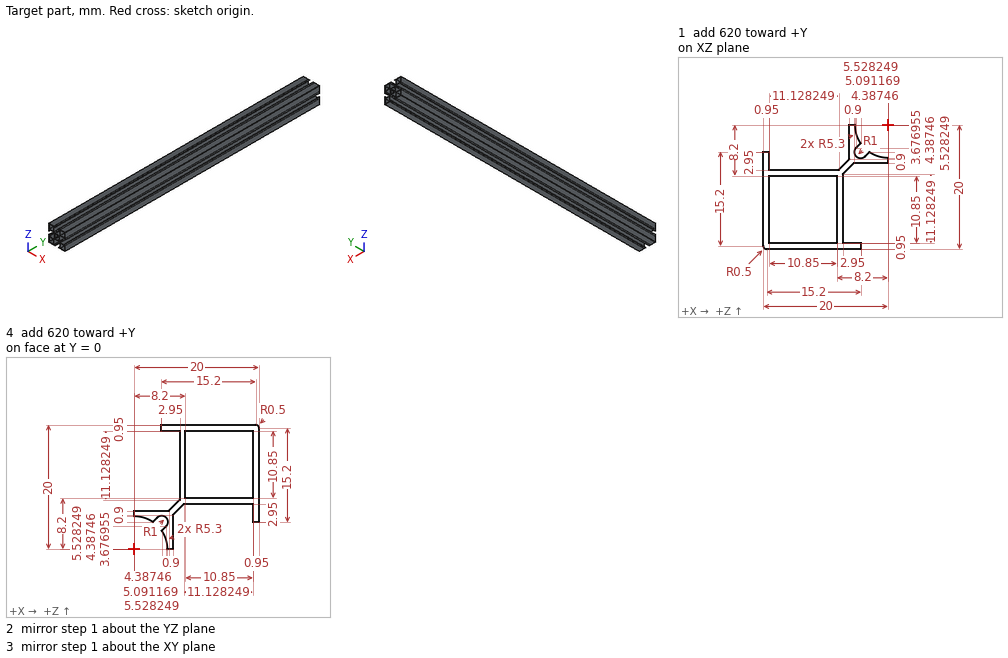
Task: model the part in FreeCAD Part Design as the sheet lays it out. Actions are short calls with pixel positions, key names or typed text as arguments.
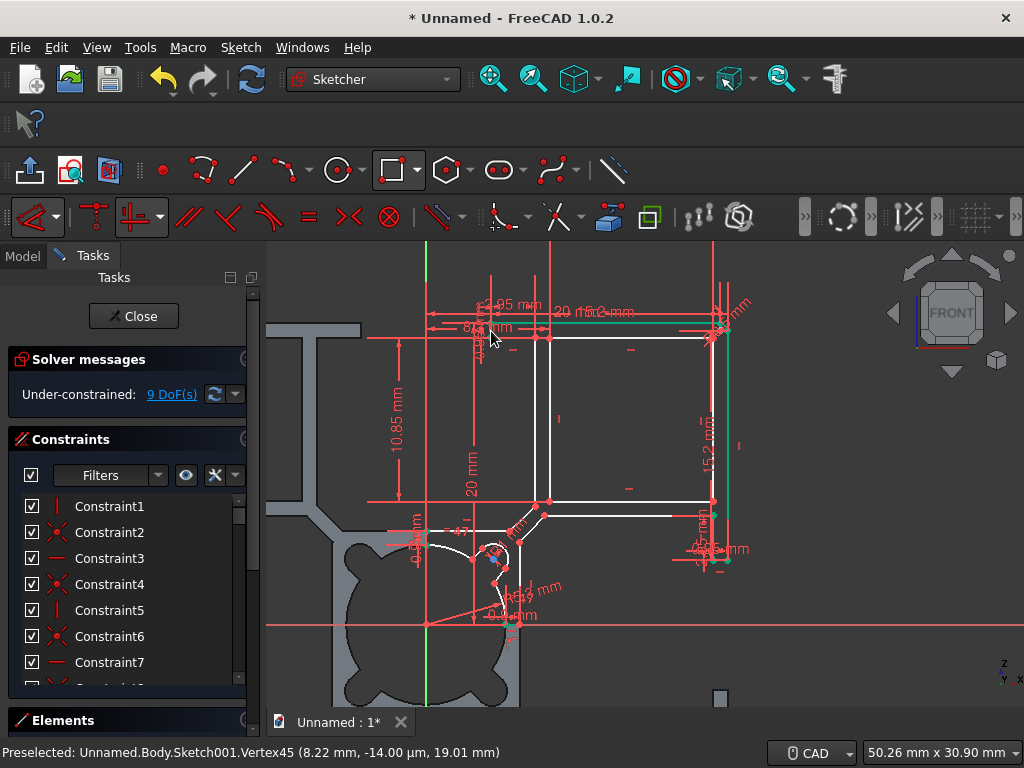
click(550, 502)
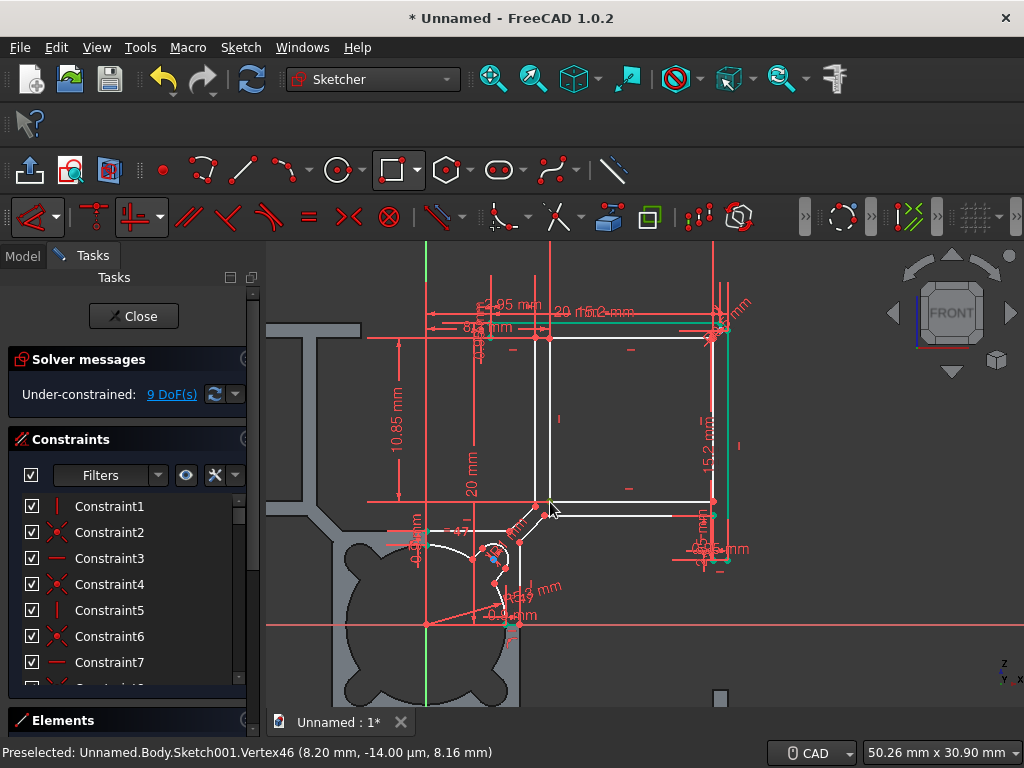
click(58, 218)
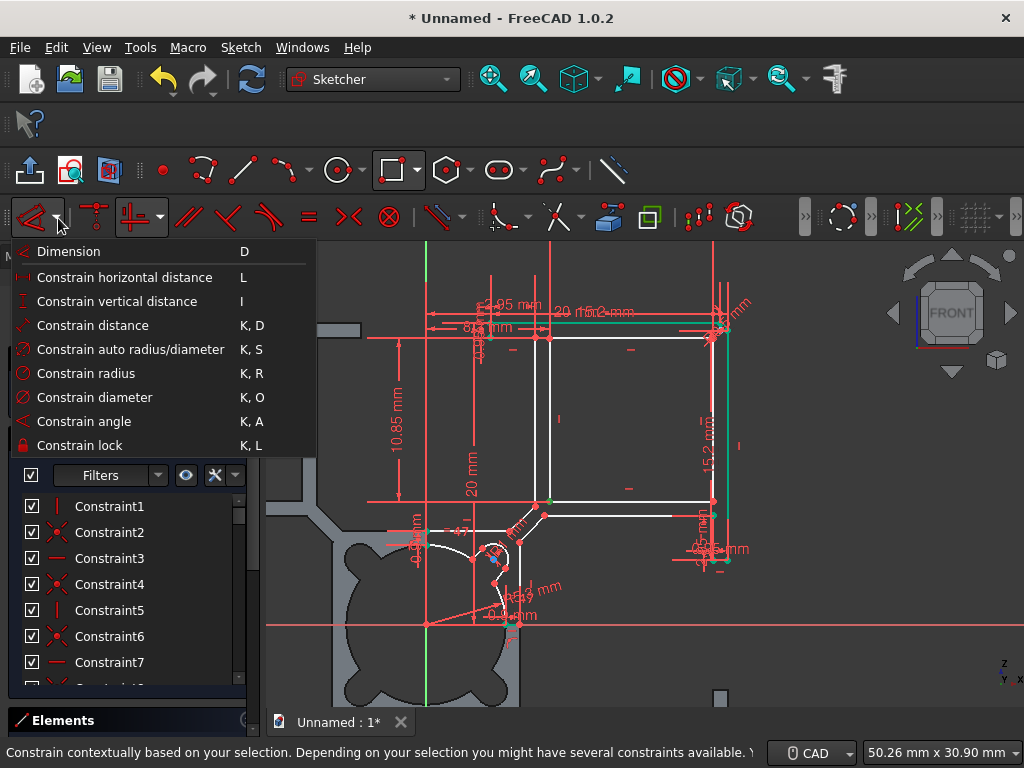
click(164, 301)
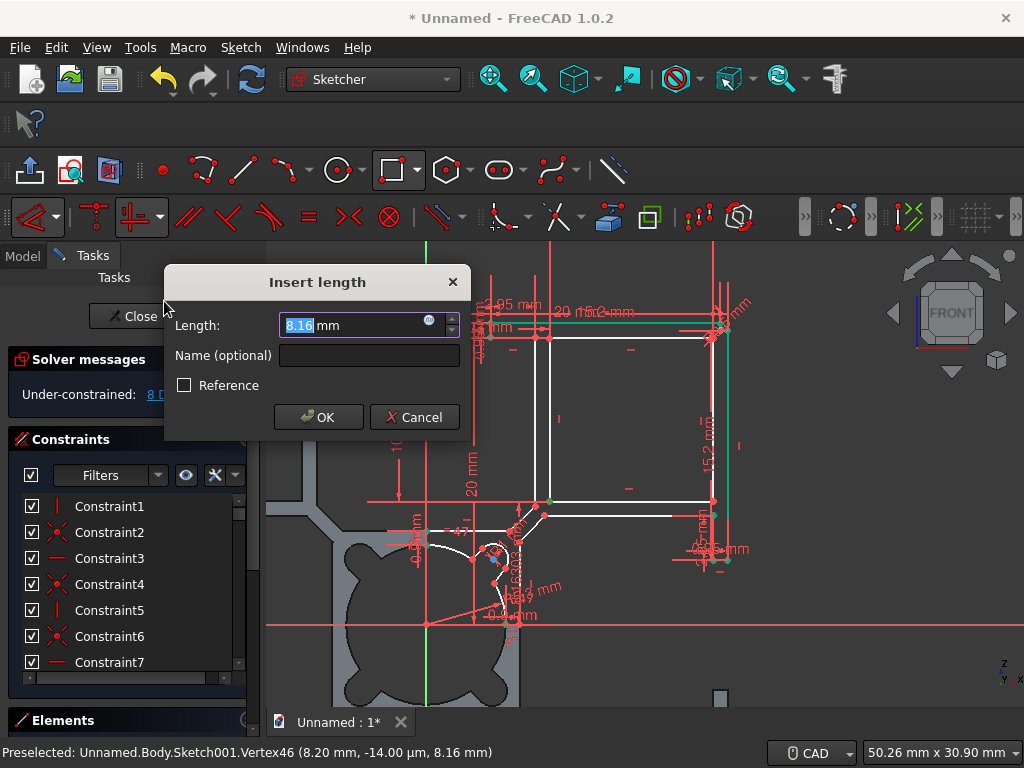
text(8.2)
key(Return)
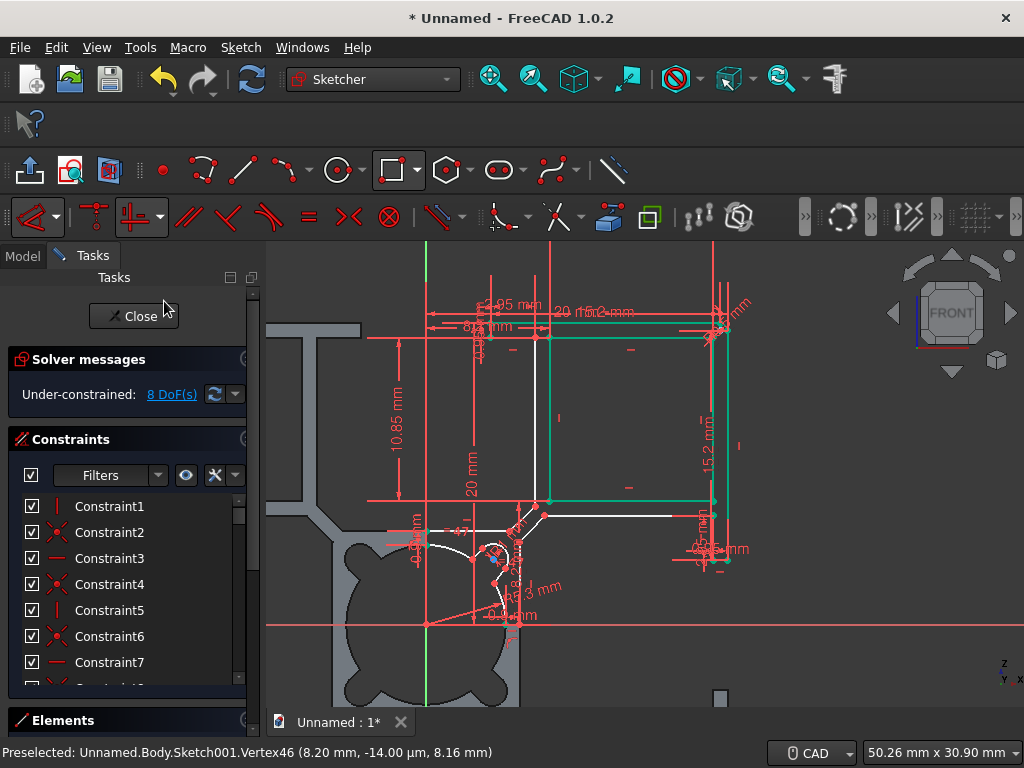
click(520, 608)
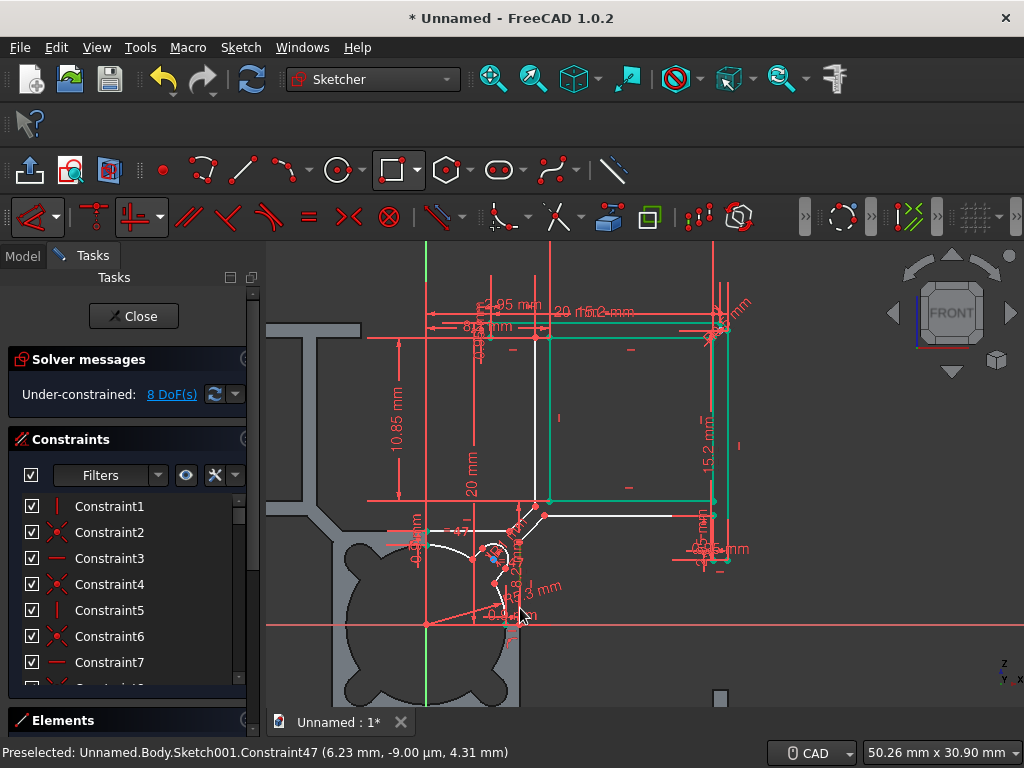
click(58, 218)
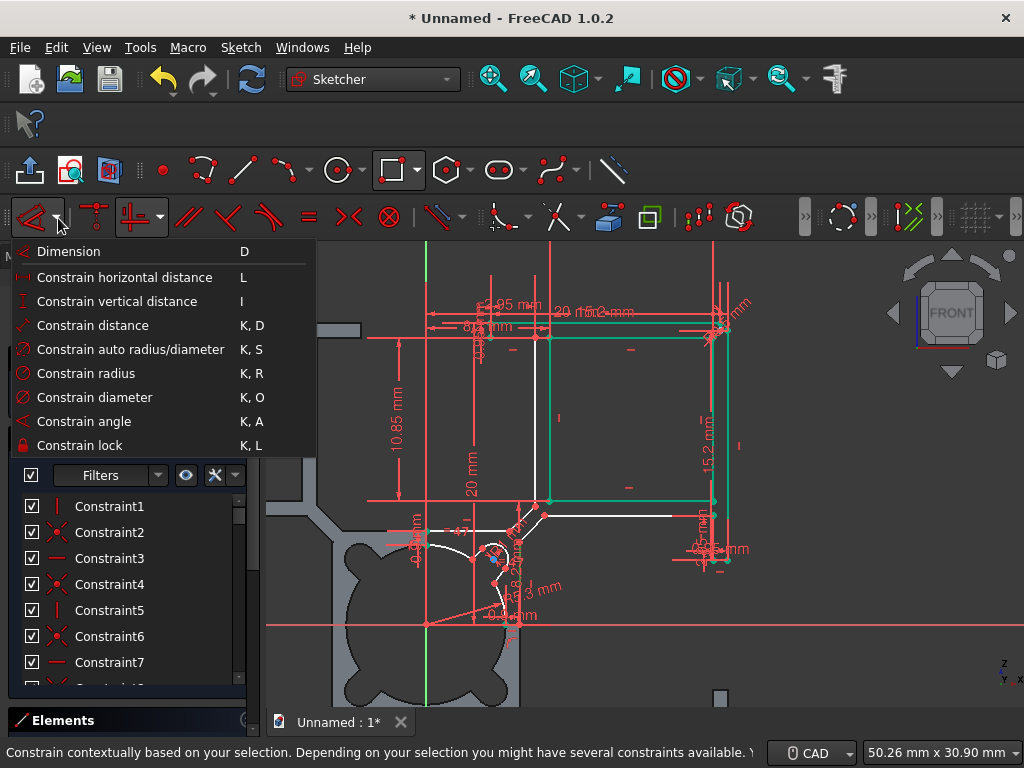
click(164, 301)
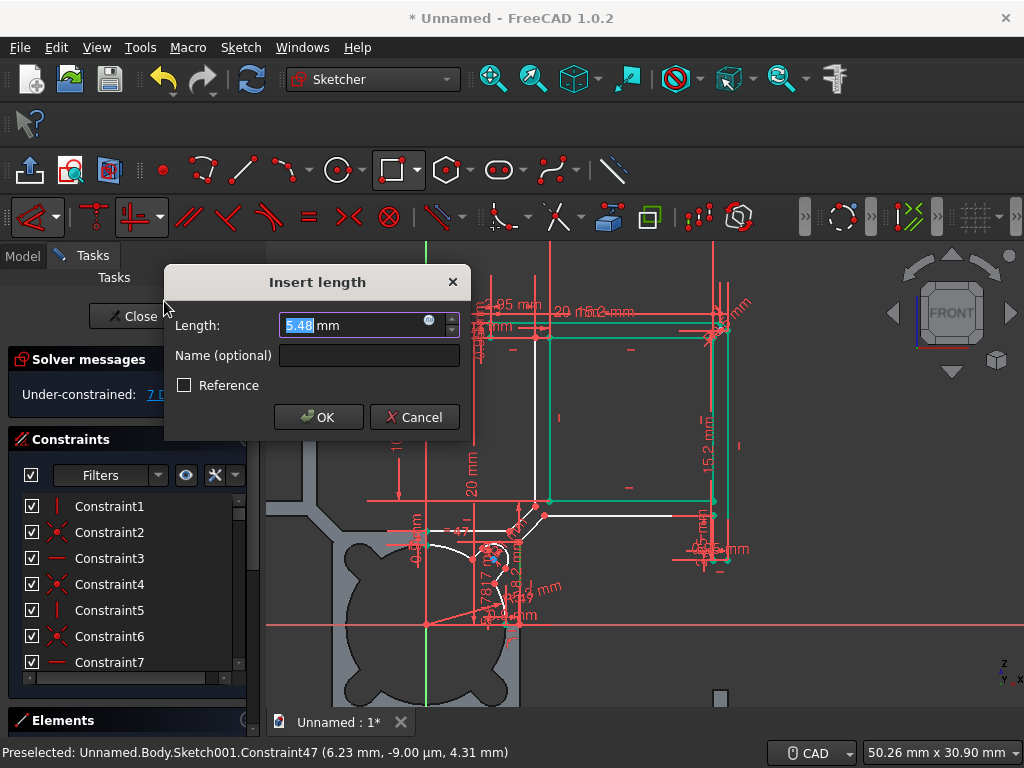
text(5.528249)
key(Return)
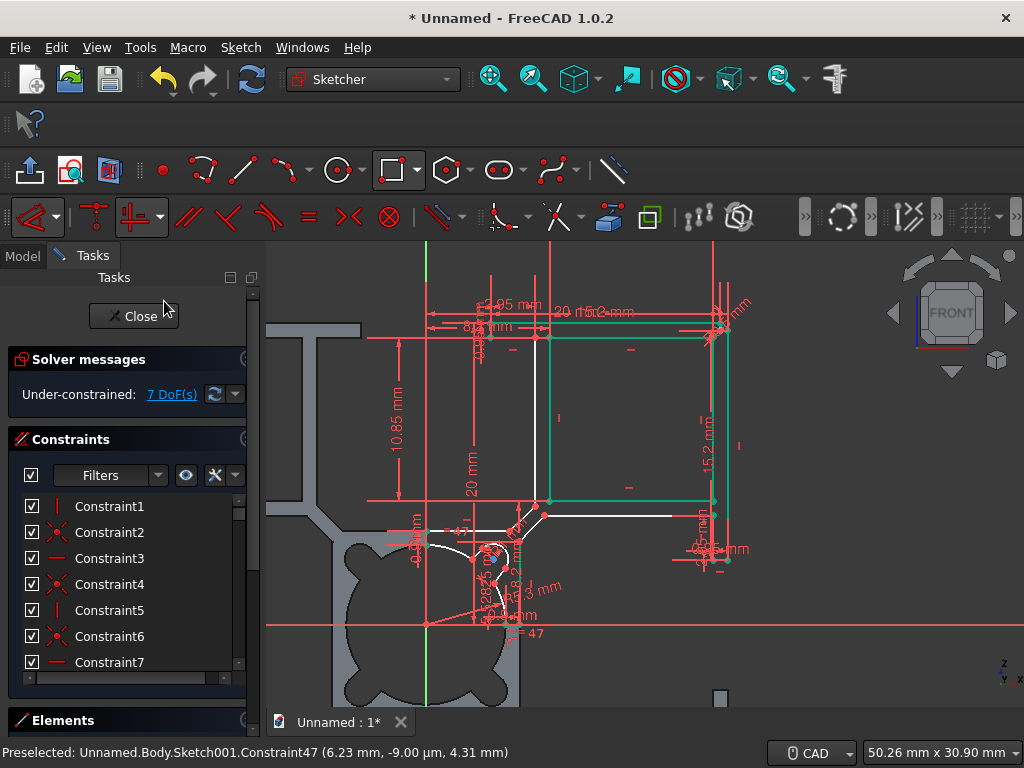
click(484, 531)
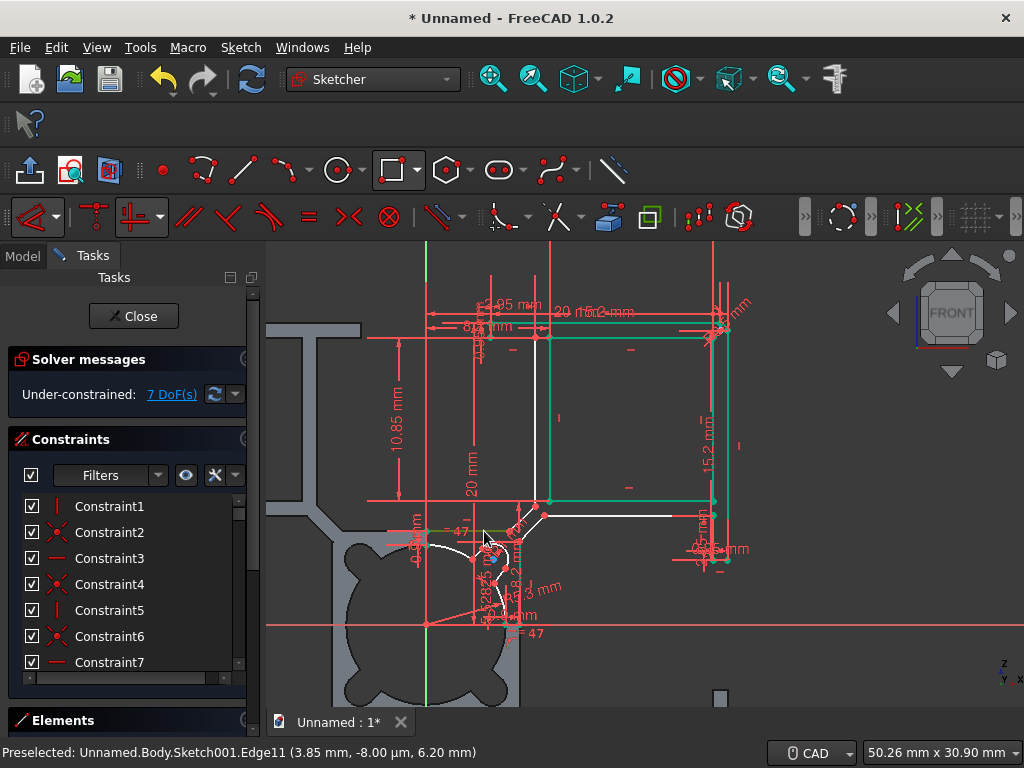
click(58, 218)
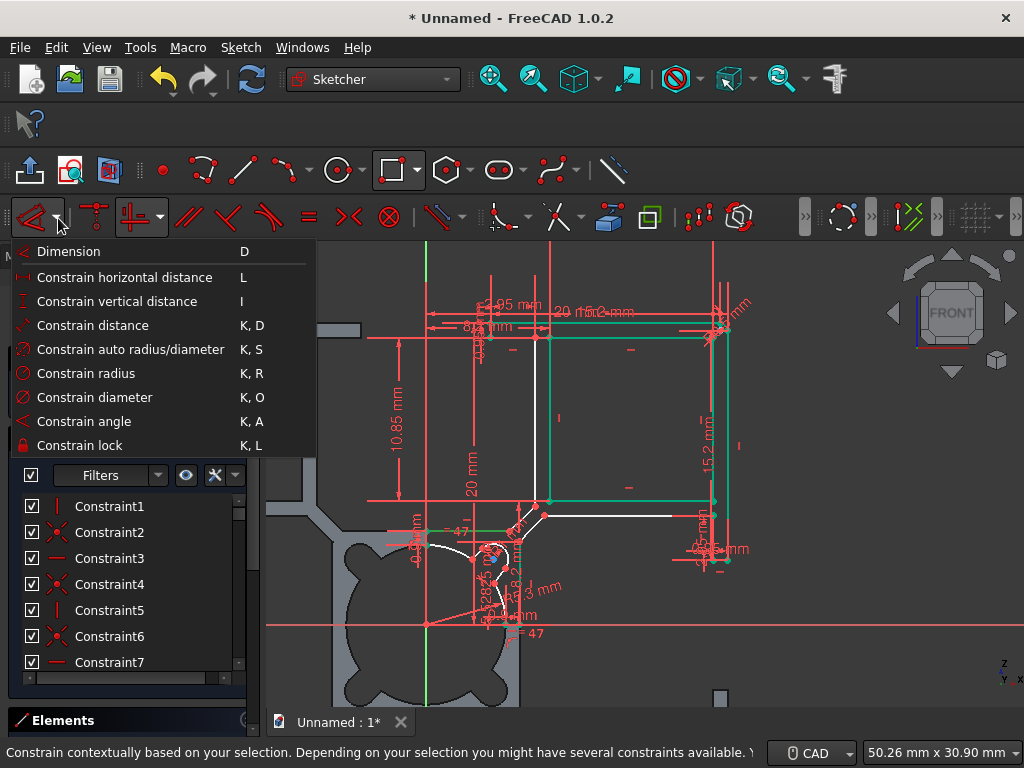
click(164, 277)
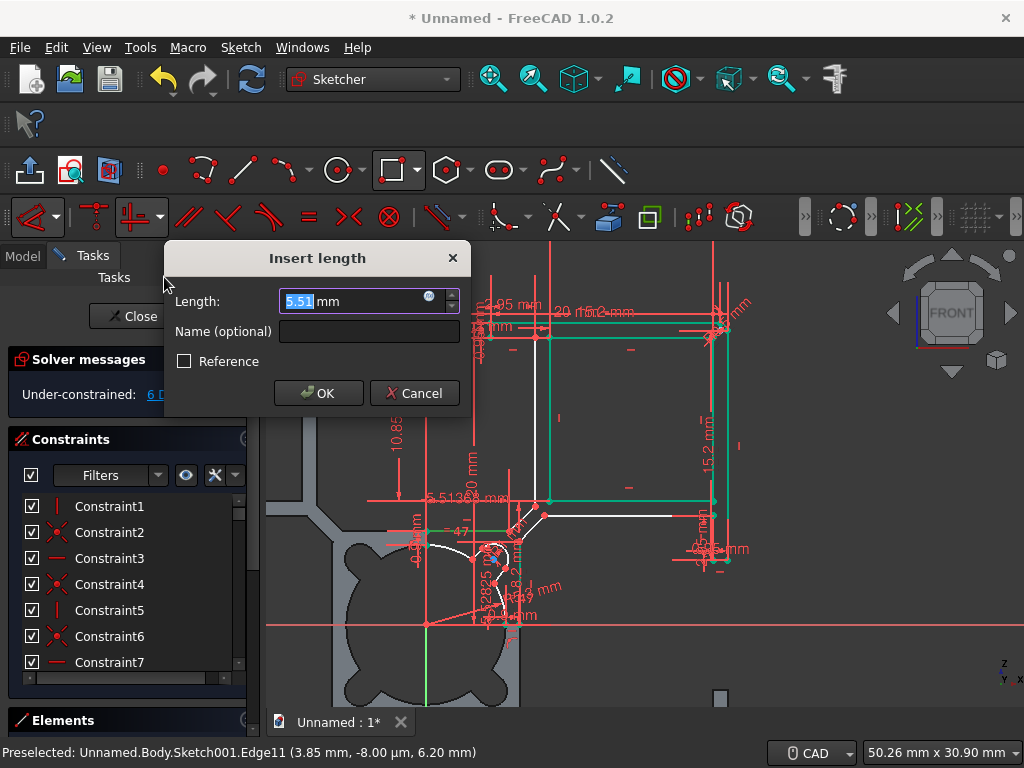
text(5.528249)
key(Return)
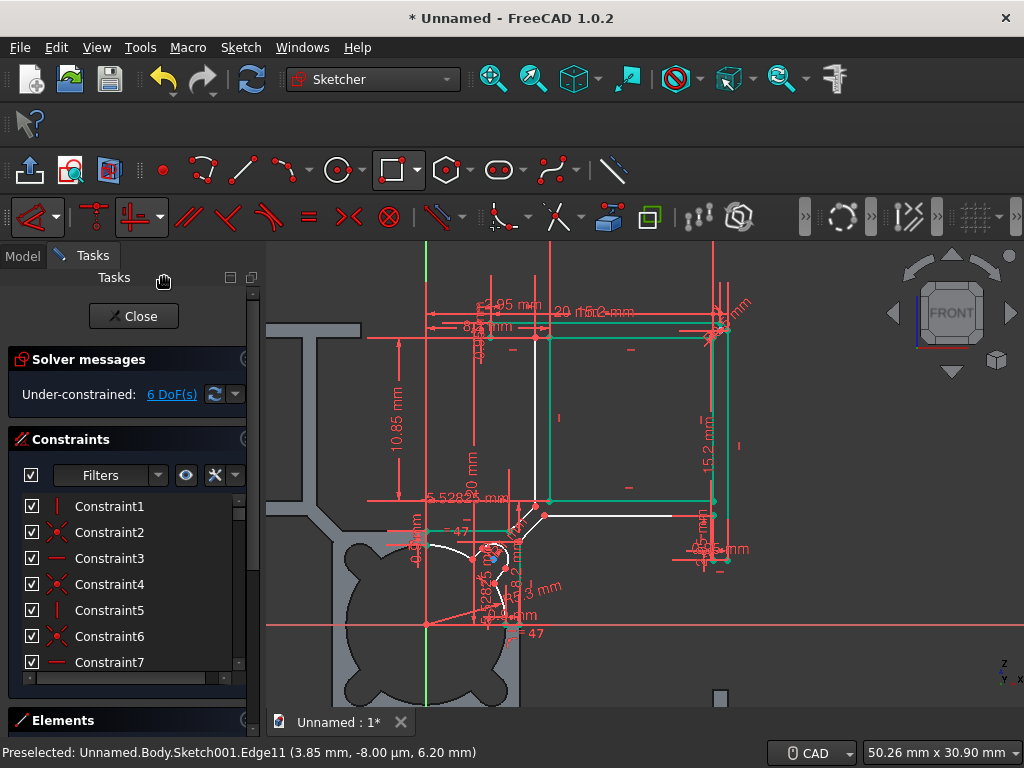
click(494, 583)